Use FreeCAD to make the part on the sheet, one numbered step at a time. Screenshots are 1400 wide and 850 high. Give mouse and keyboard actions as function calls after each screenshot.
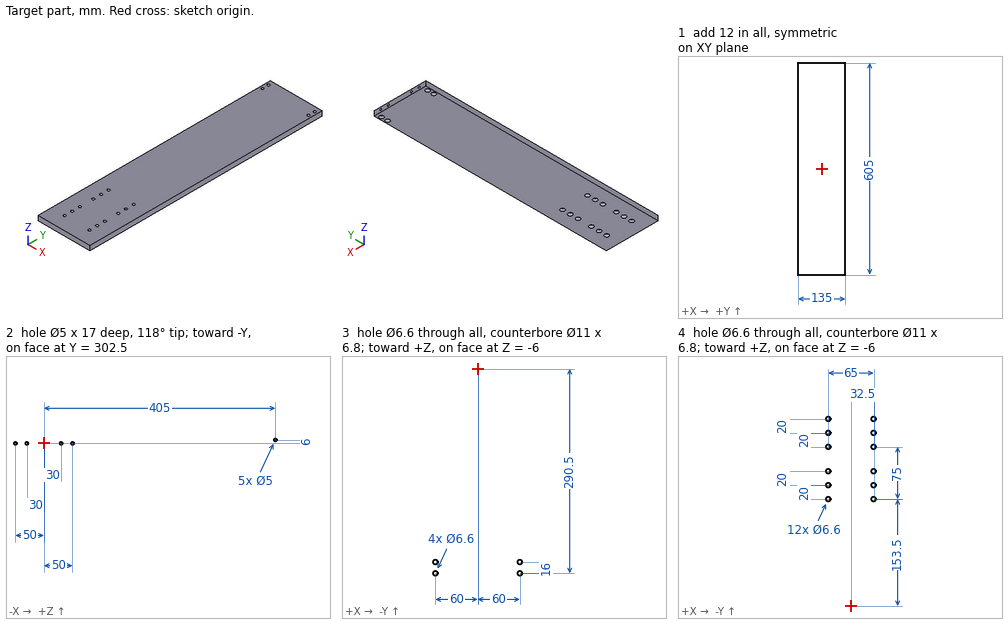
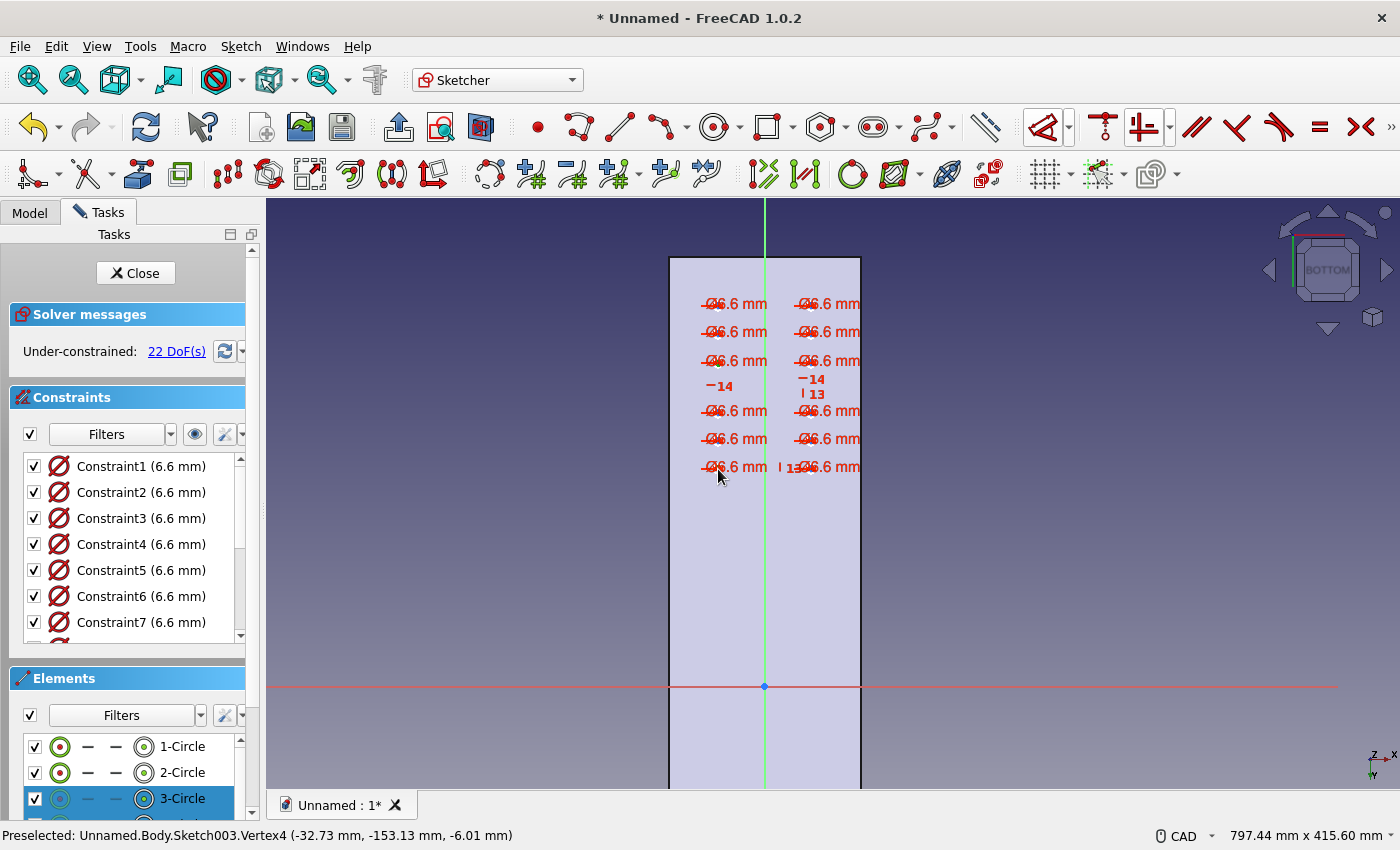
click(1170, 128)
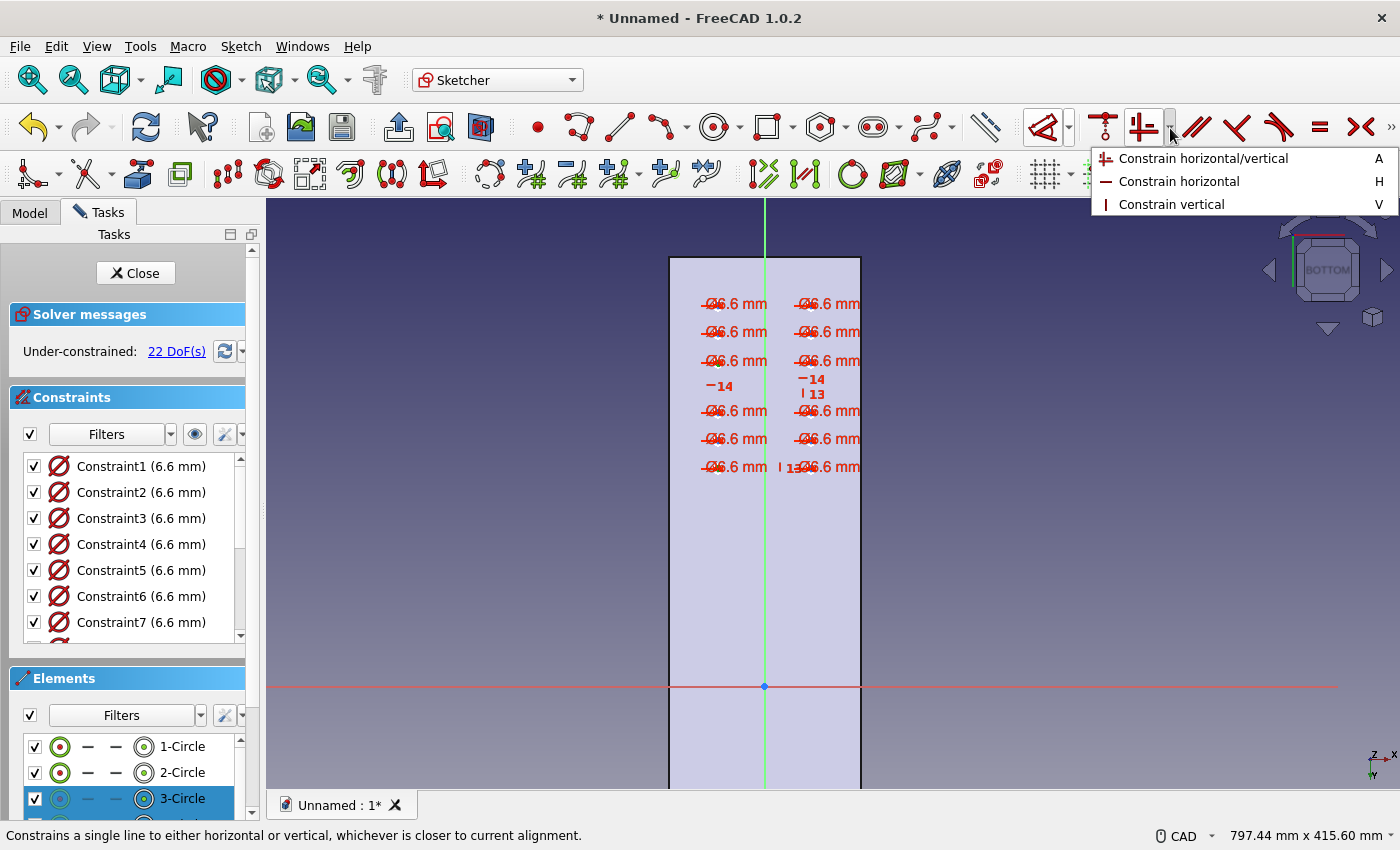
click(1245, 204)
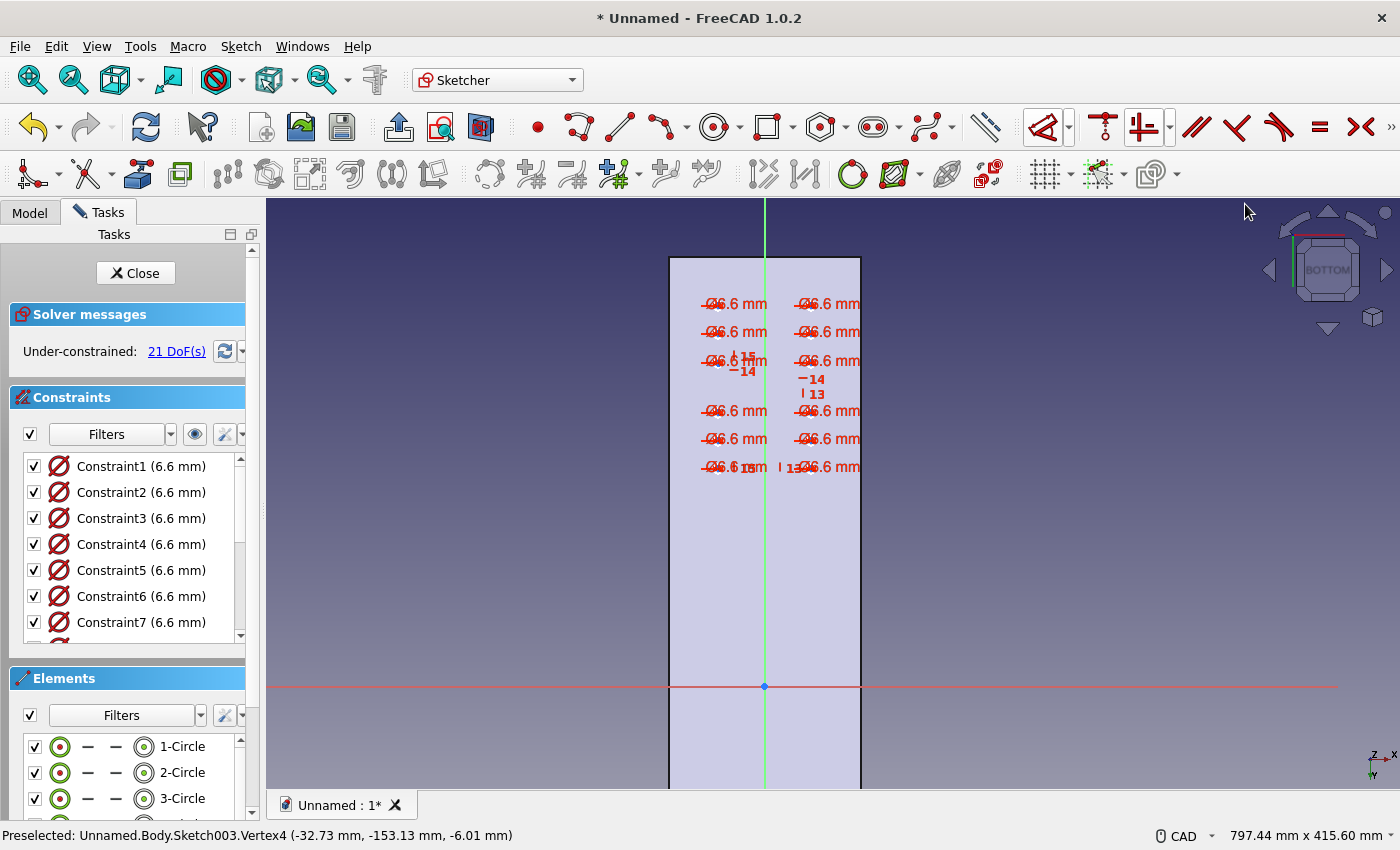
click(811, 469)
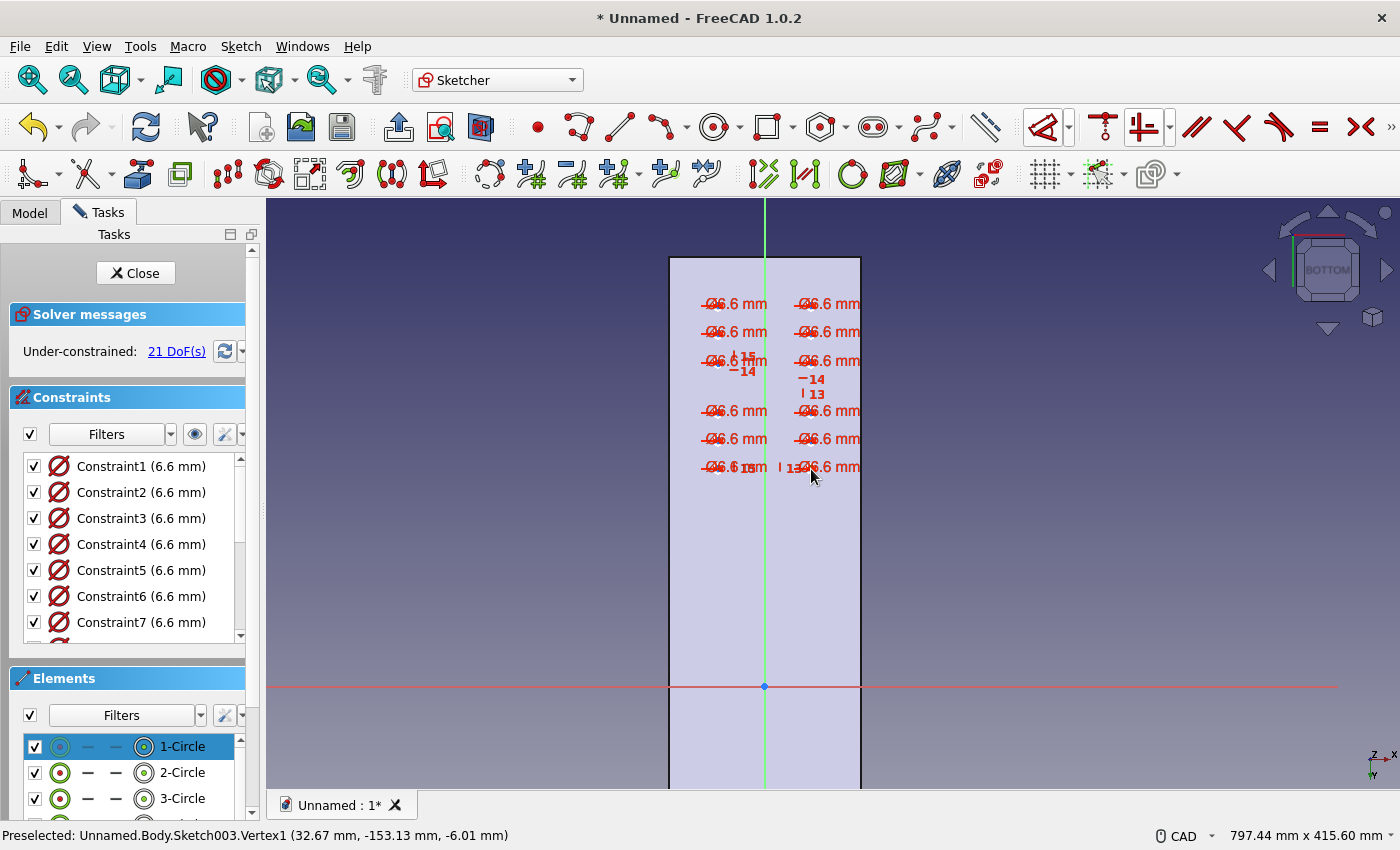
click(718, 469)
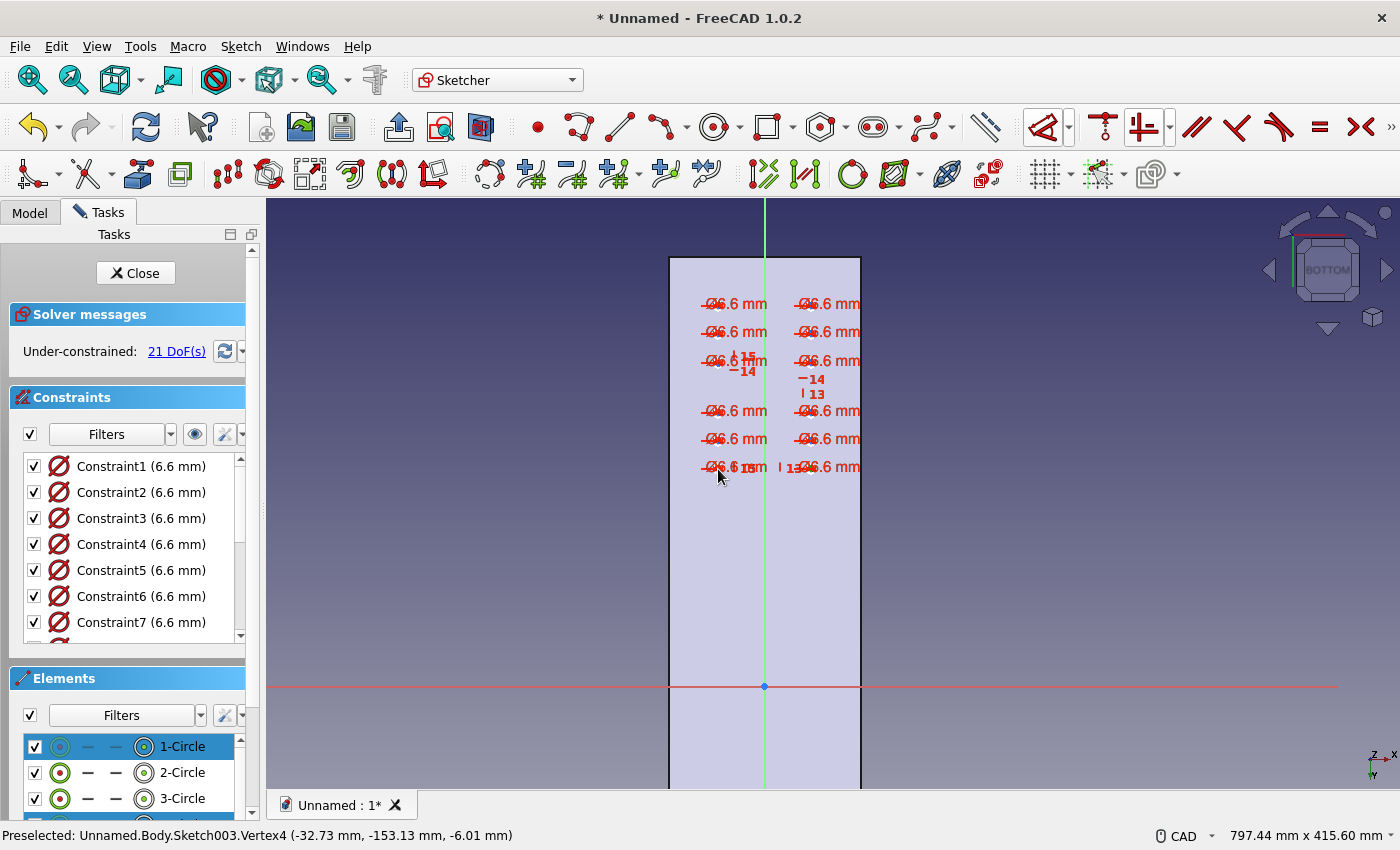
key(h)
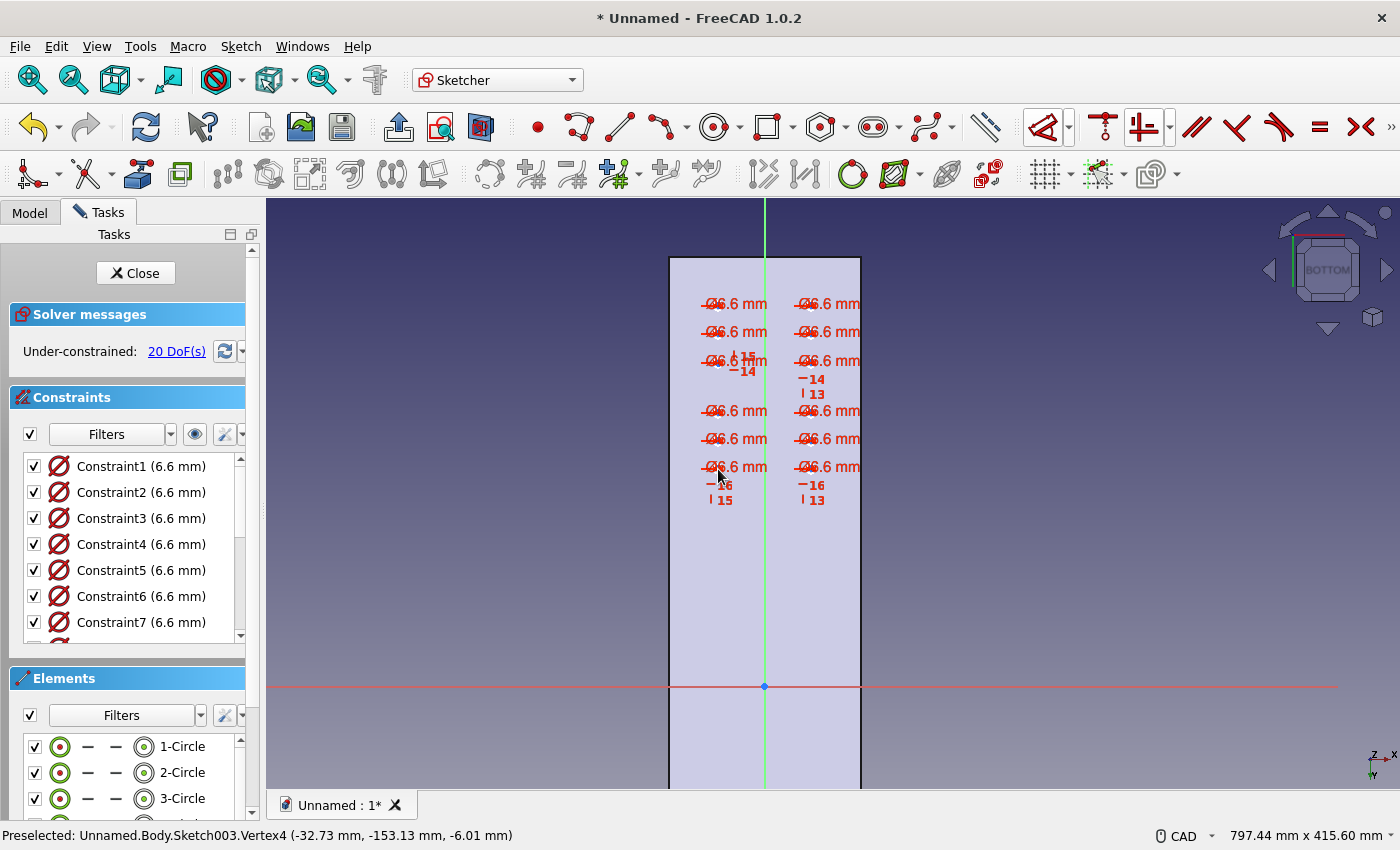
click(718, 469)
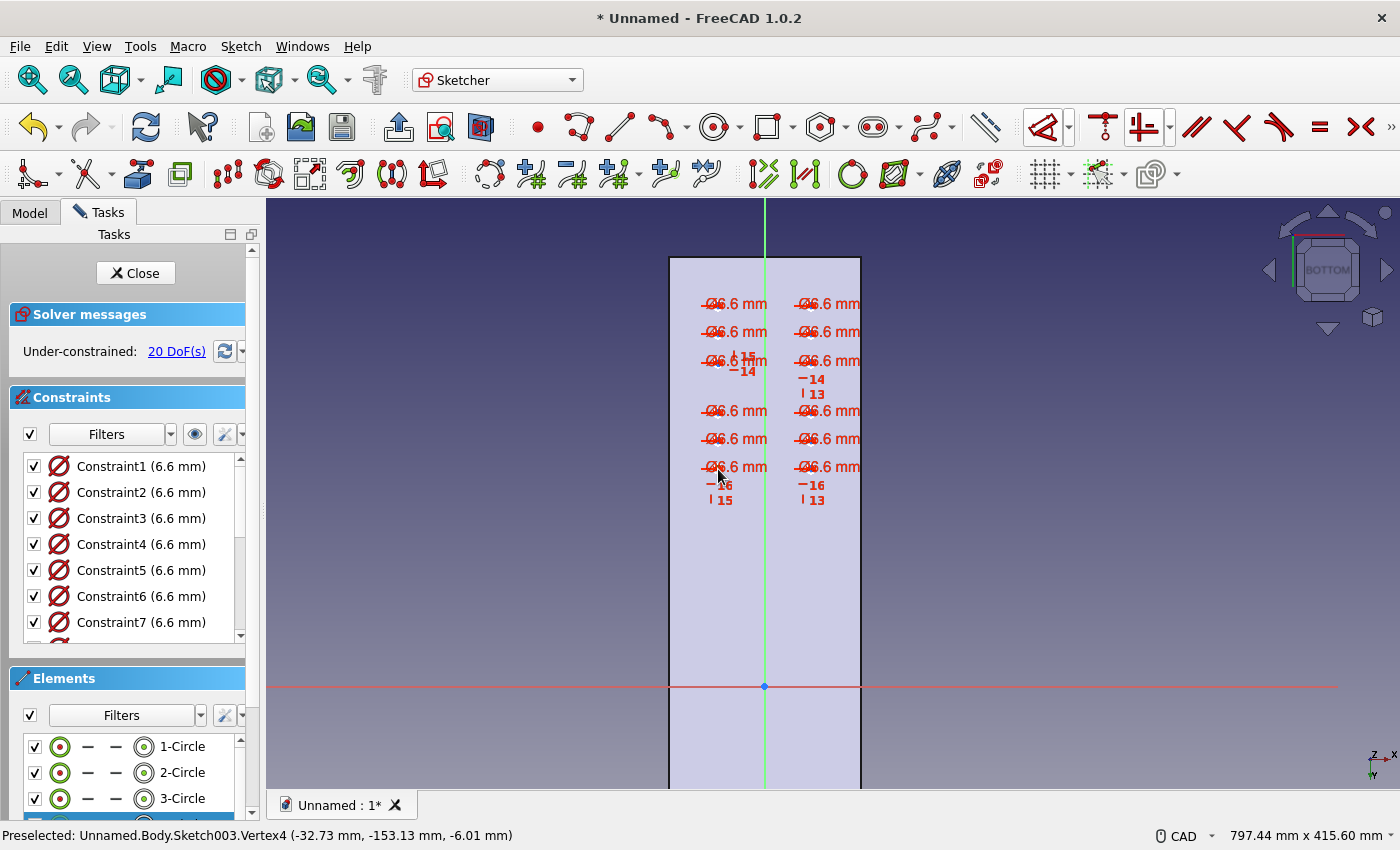
click(718, 441)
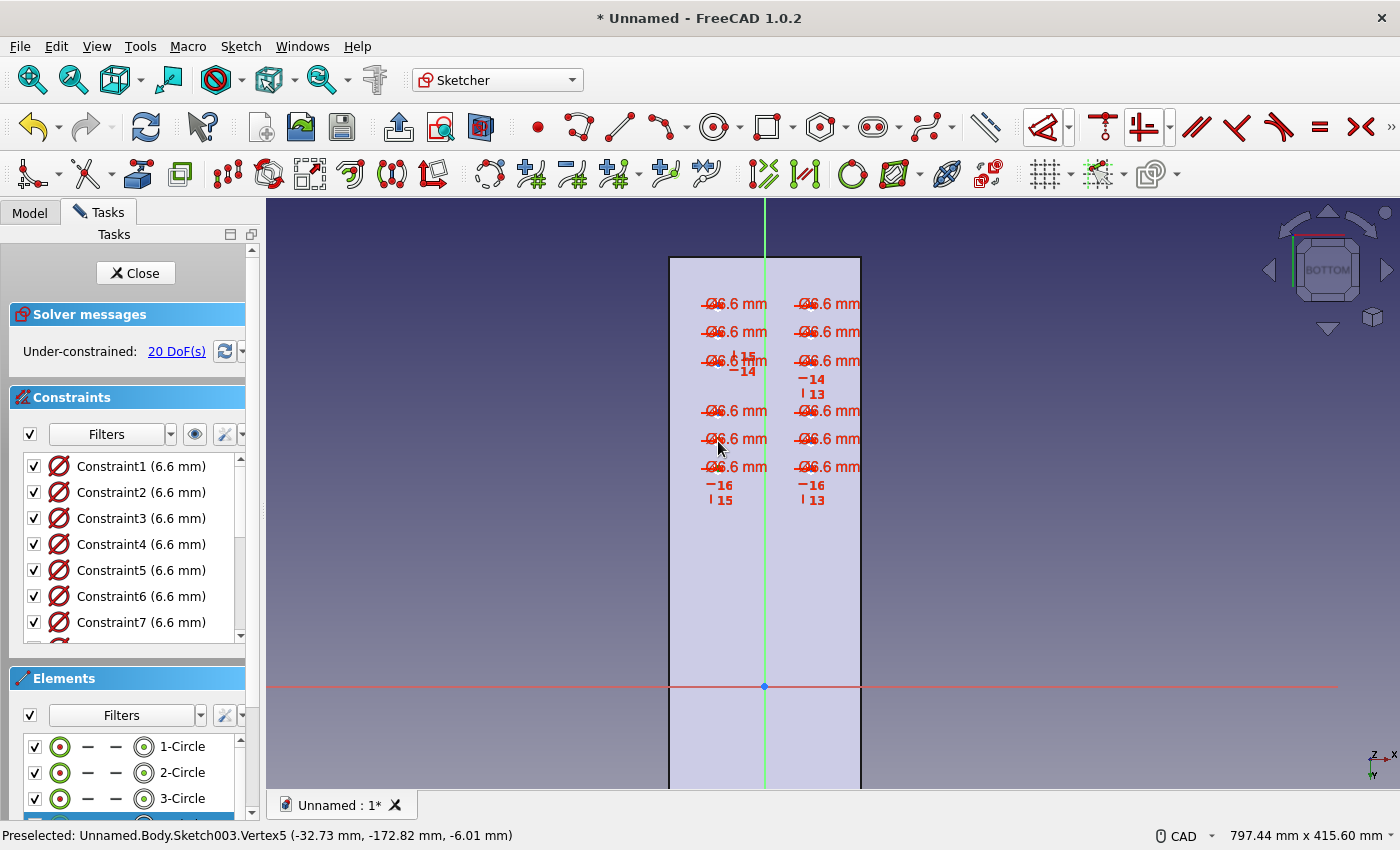
click(1170, 128)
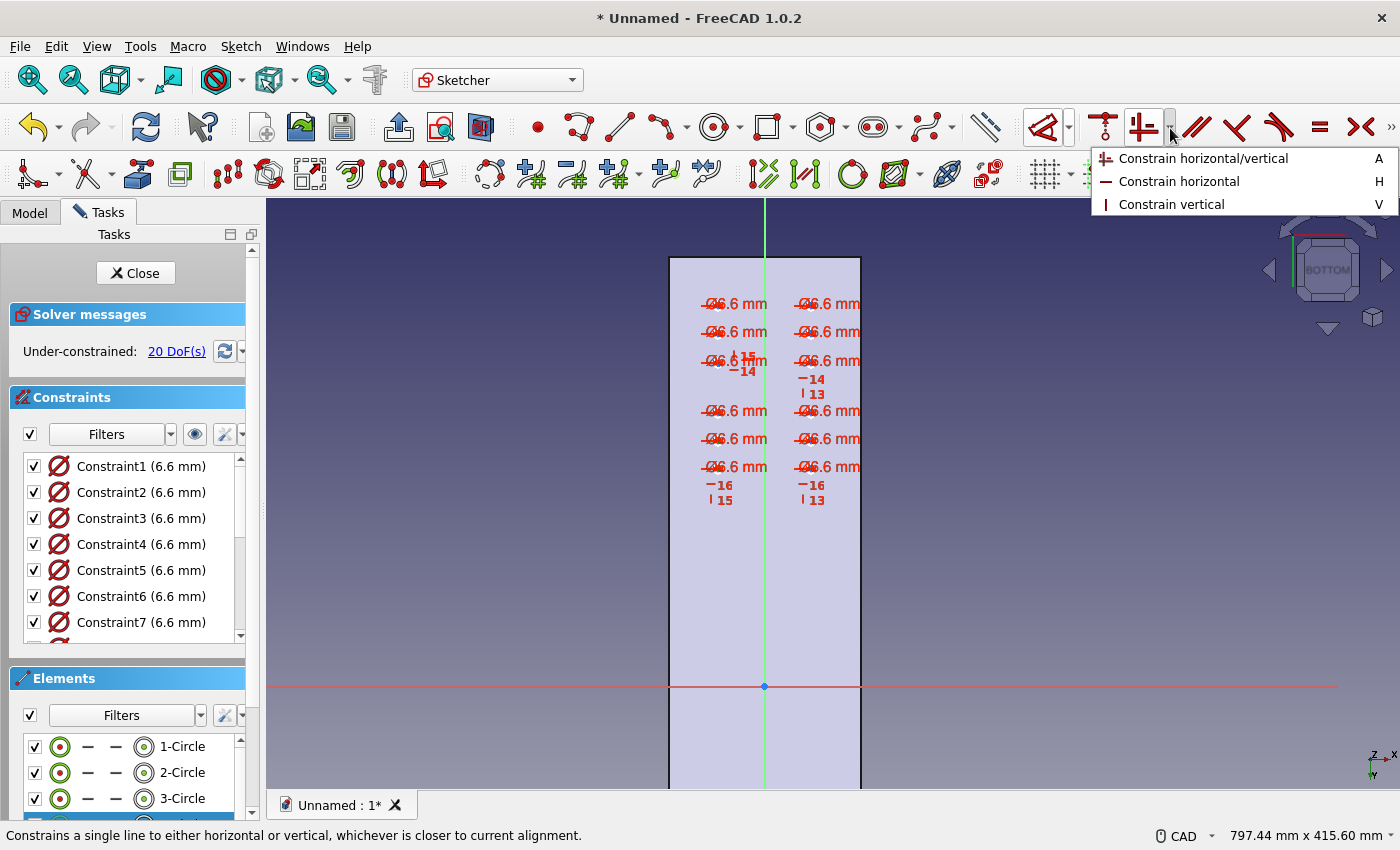
click(1245, 204)